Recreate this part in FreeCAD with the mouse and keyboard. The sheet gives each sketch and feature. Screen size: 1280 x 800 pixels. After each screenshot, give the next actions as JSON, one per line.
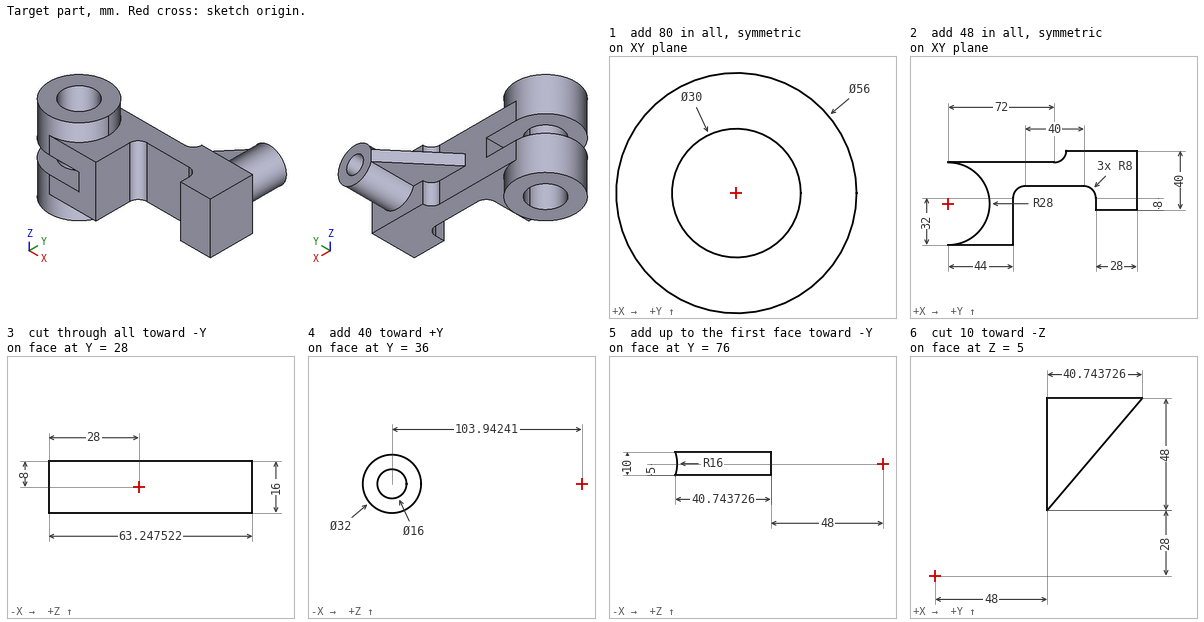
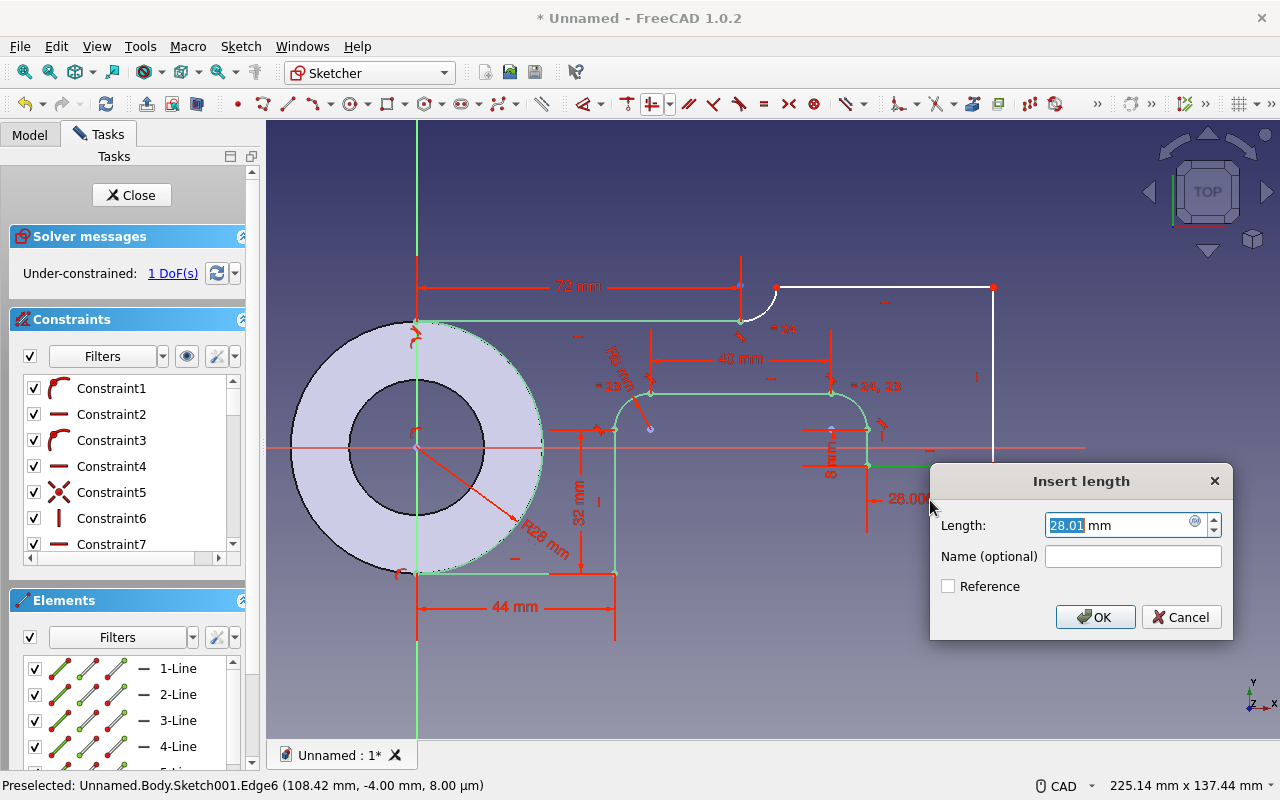
{"action": "type", "text": "28"}
{"action": "key", "text": "Return"}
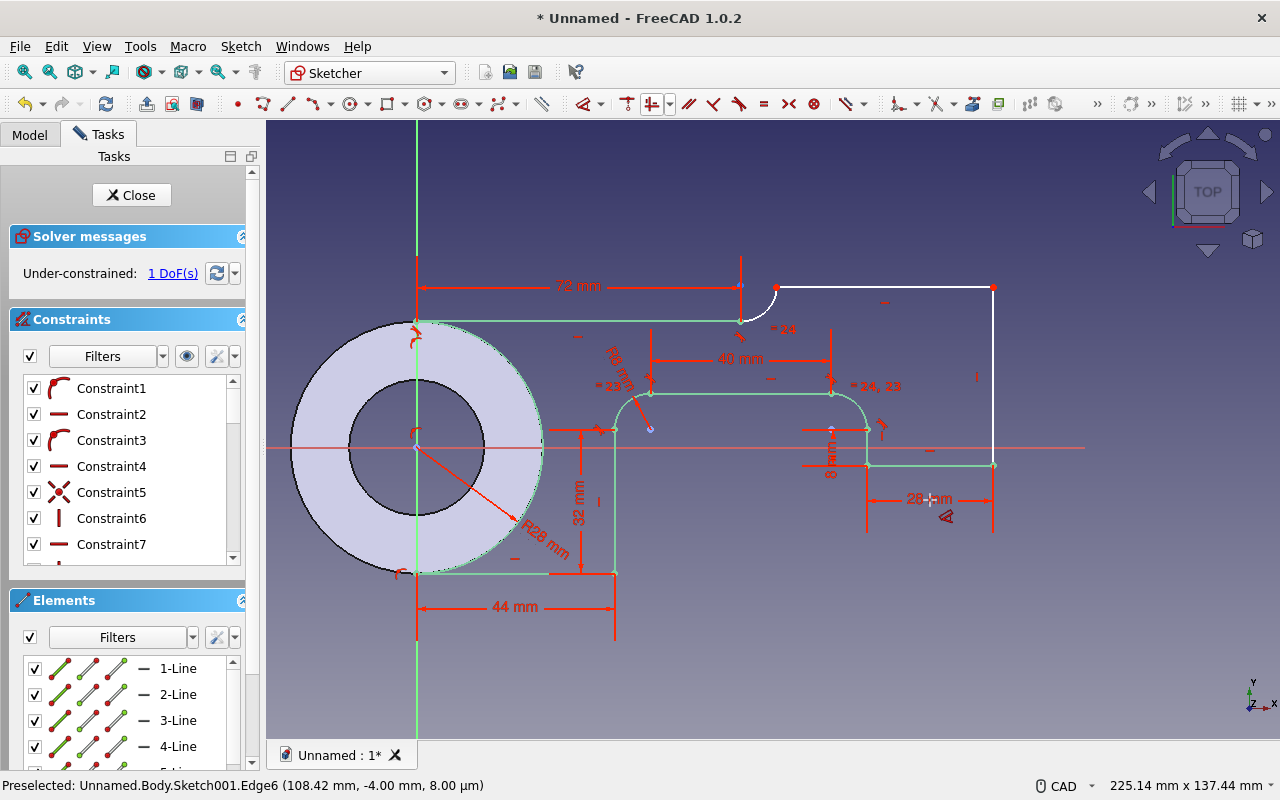
{"action": "left_click", "coordinate": [993, 412]}
{"action": "left_click", "coordinate": [1027, 376]}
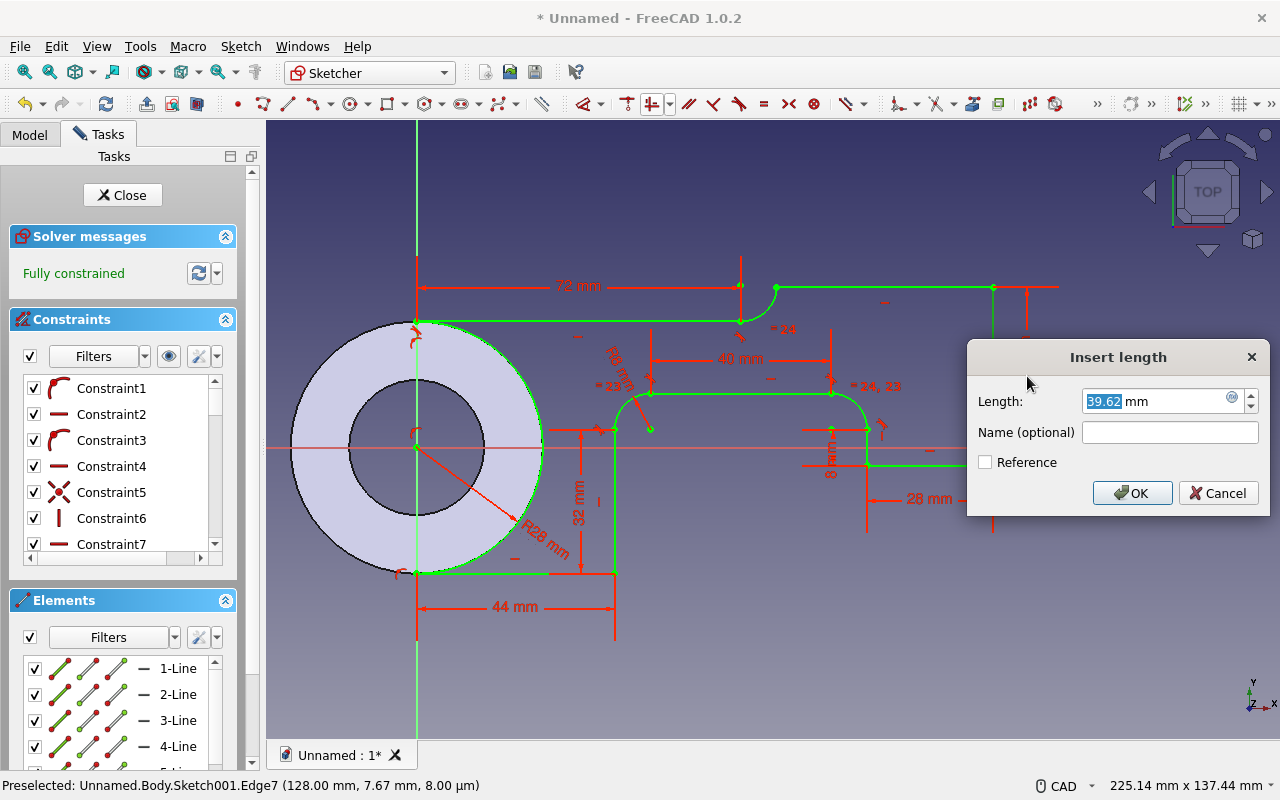
{"action": "type", "text": "40"}
{"action": "key", "text": "Return"}
{"action": "key", "text": "Escape"}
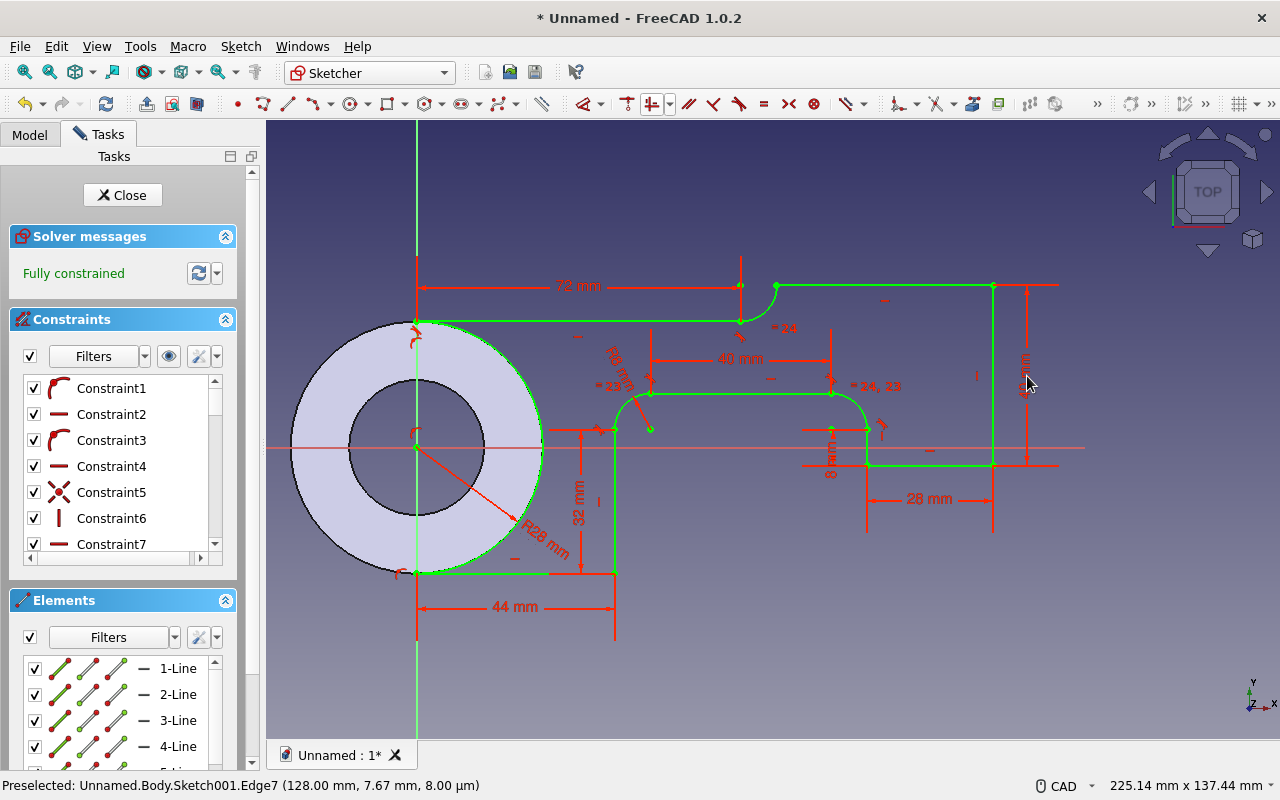
{"action": "left_click", "coordinate": [123, 195]}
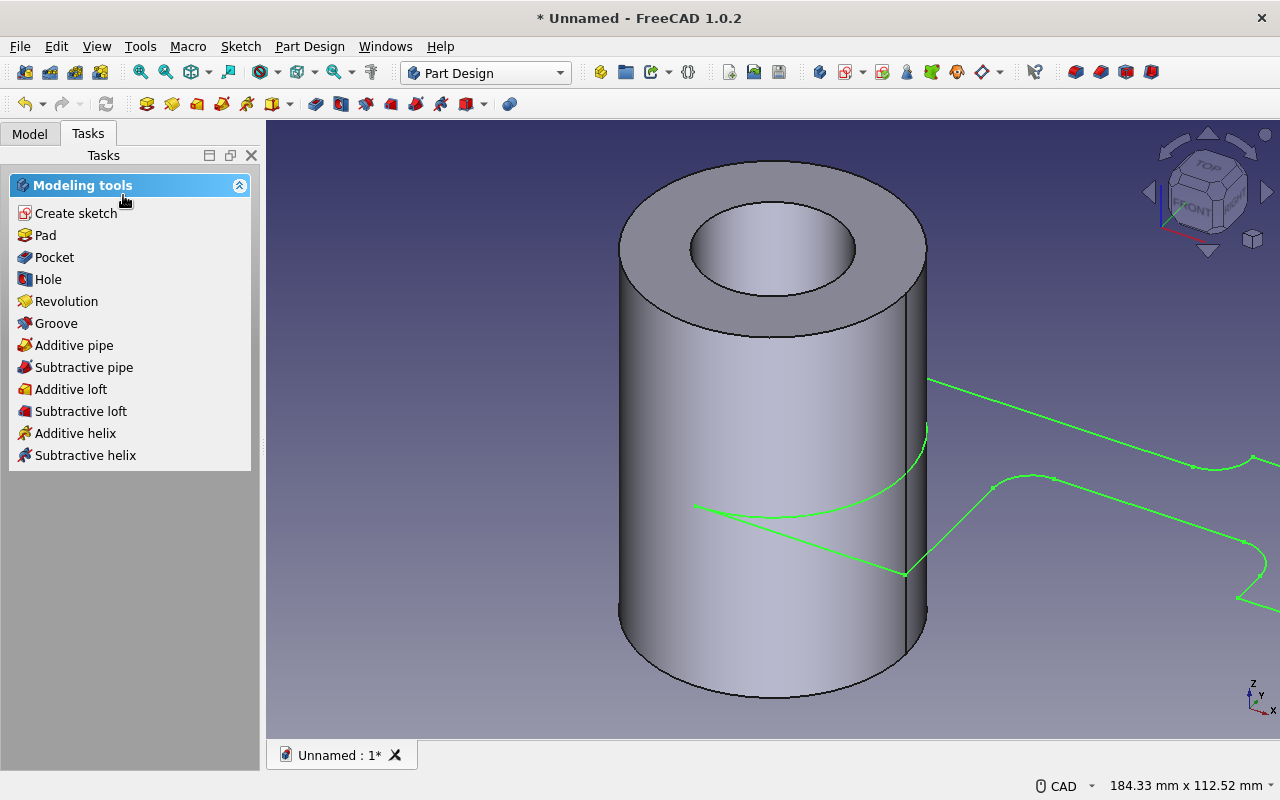
{"action": "left_click", "coordinate": [147, 104]}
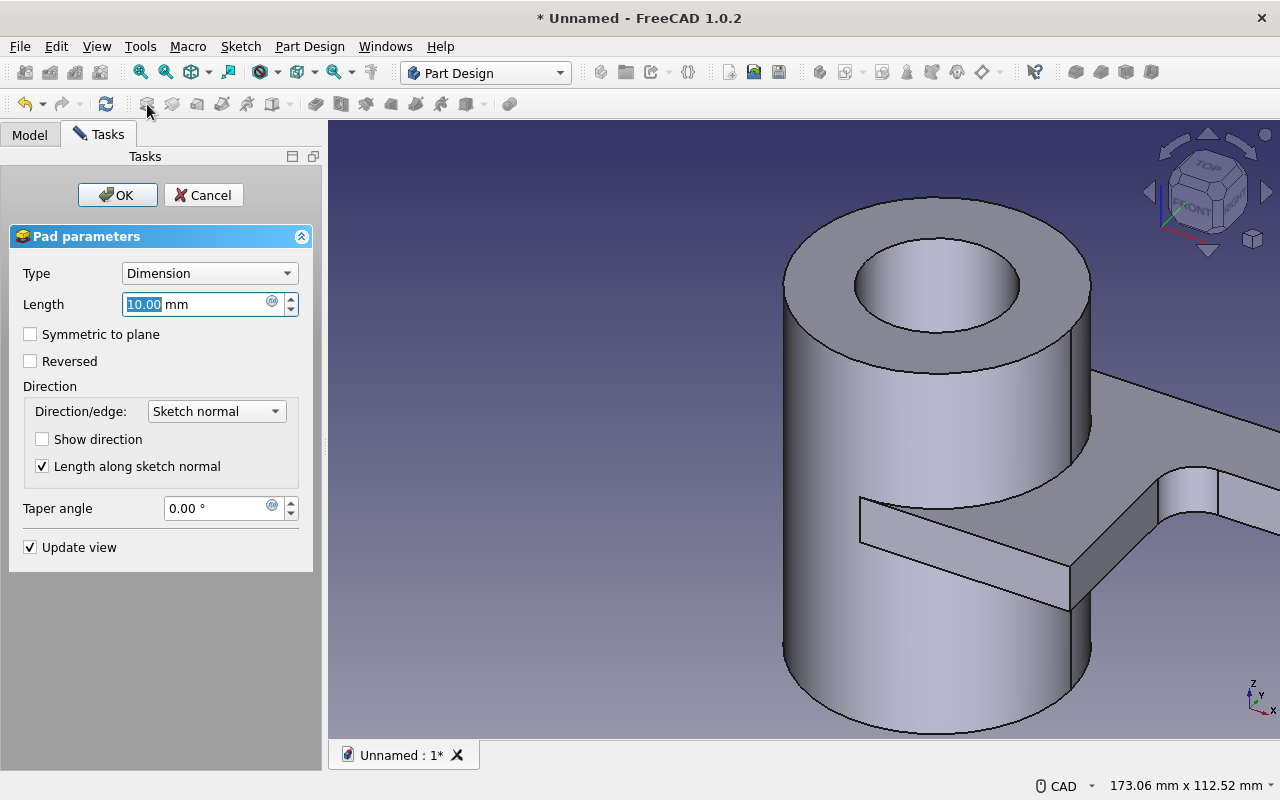
{"action": "type", "text": "48"}
{"action": "key", "text": "Tab"}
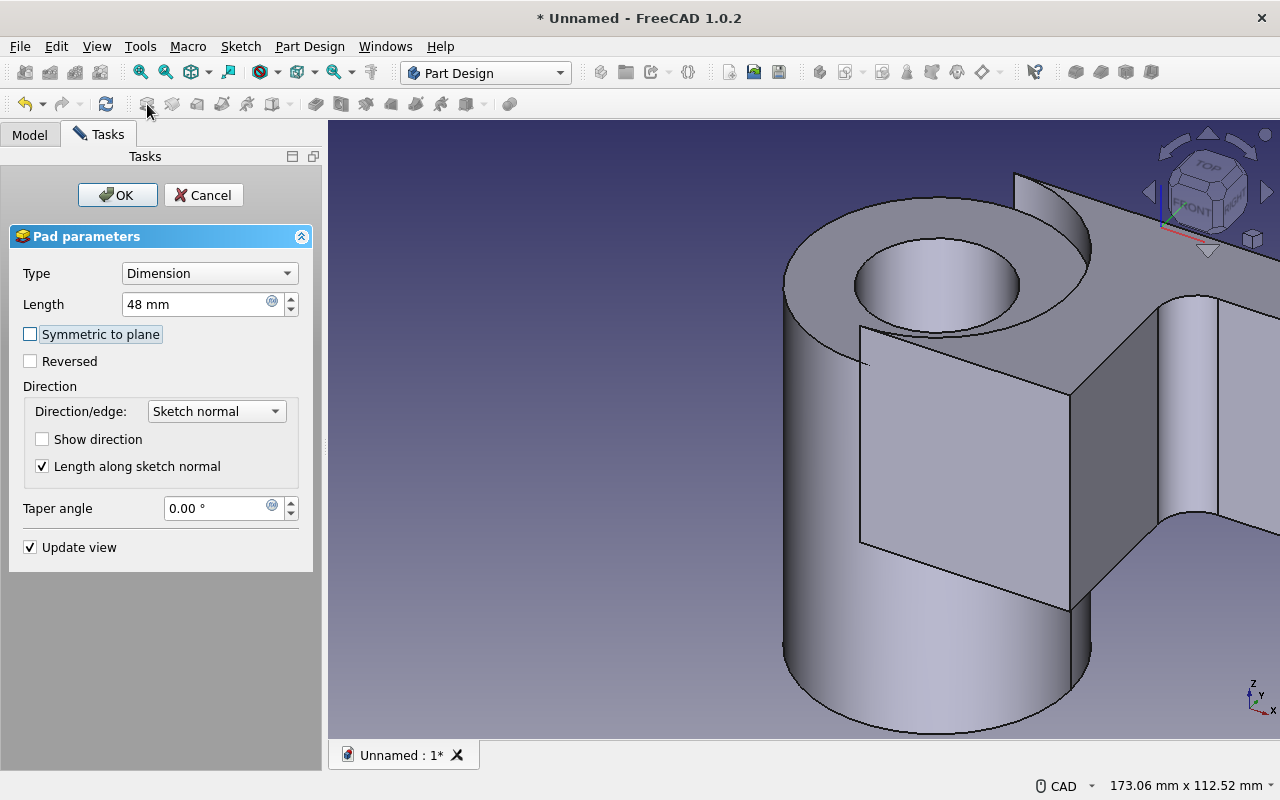
{"action": "left_click", "coordinate": [31, 334]}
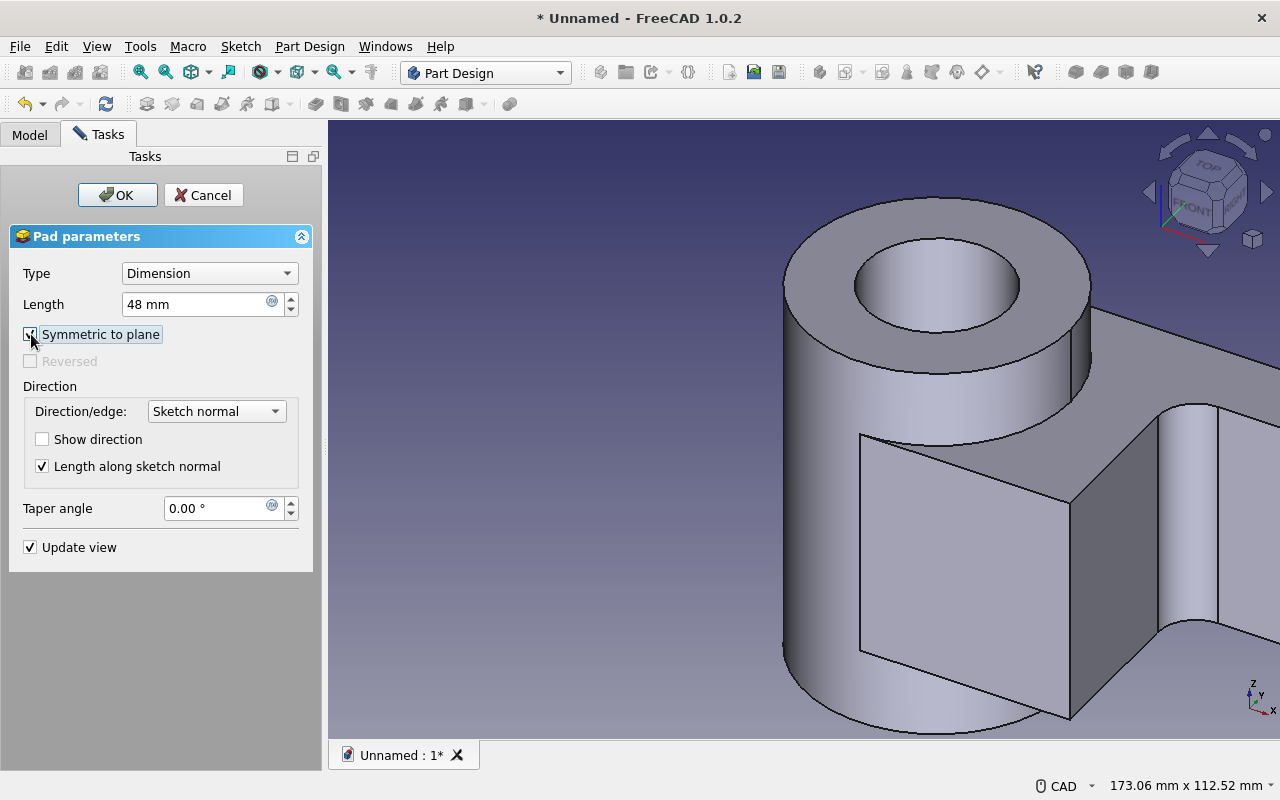
{"action": "left_click", "coordinate": [118, 195]}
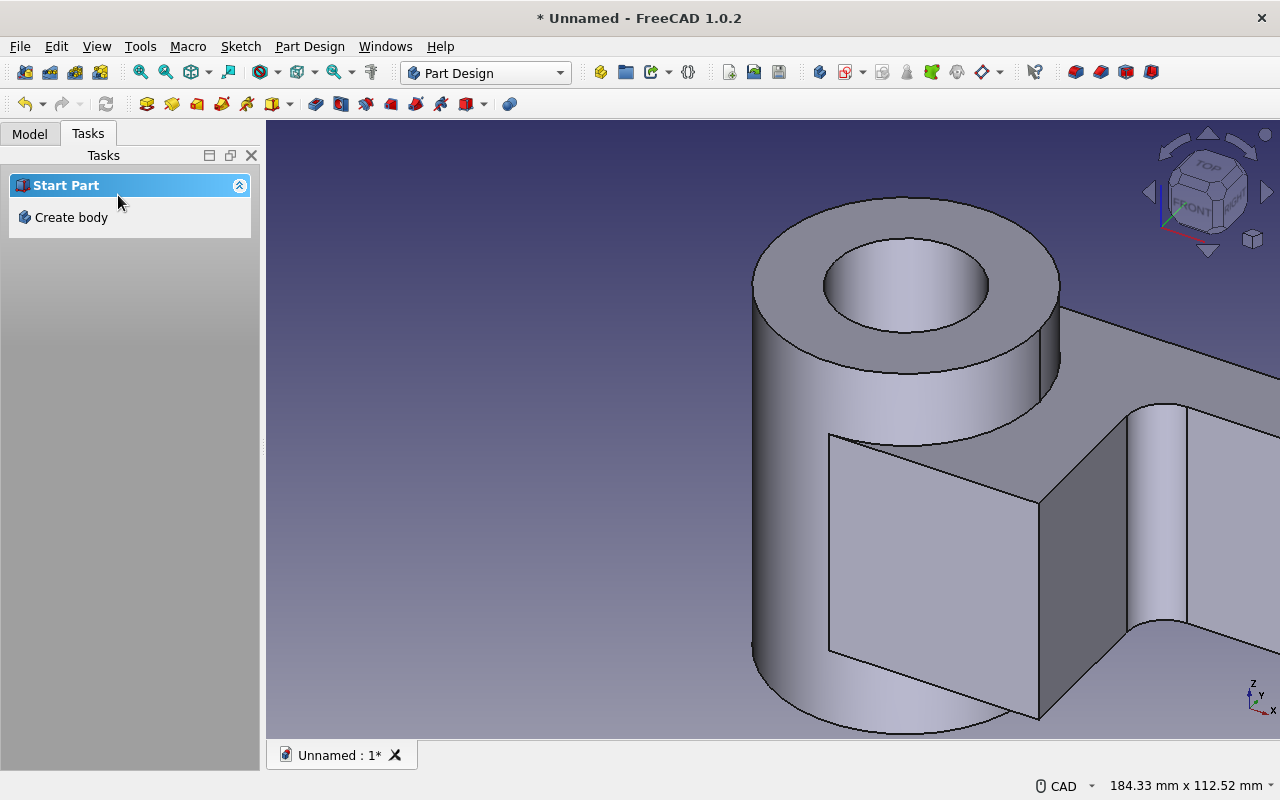
{"action": "left_click", "coordinate": [141, 72]}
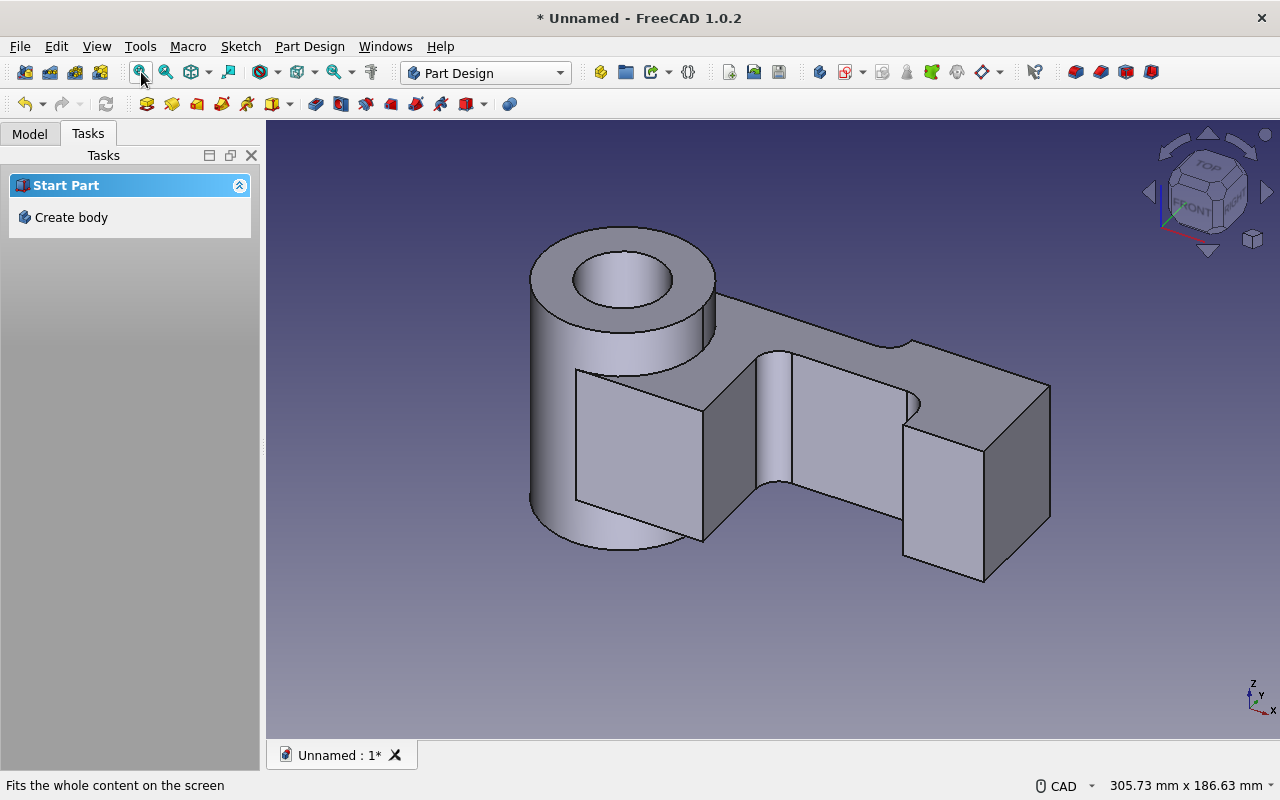
{"action": "key", "text": "4"}